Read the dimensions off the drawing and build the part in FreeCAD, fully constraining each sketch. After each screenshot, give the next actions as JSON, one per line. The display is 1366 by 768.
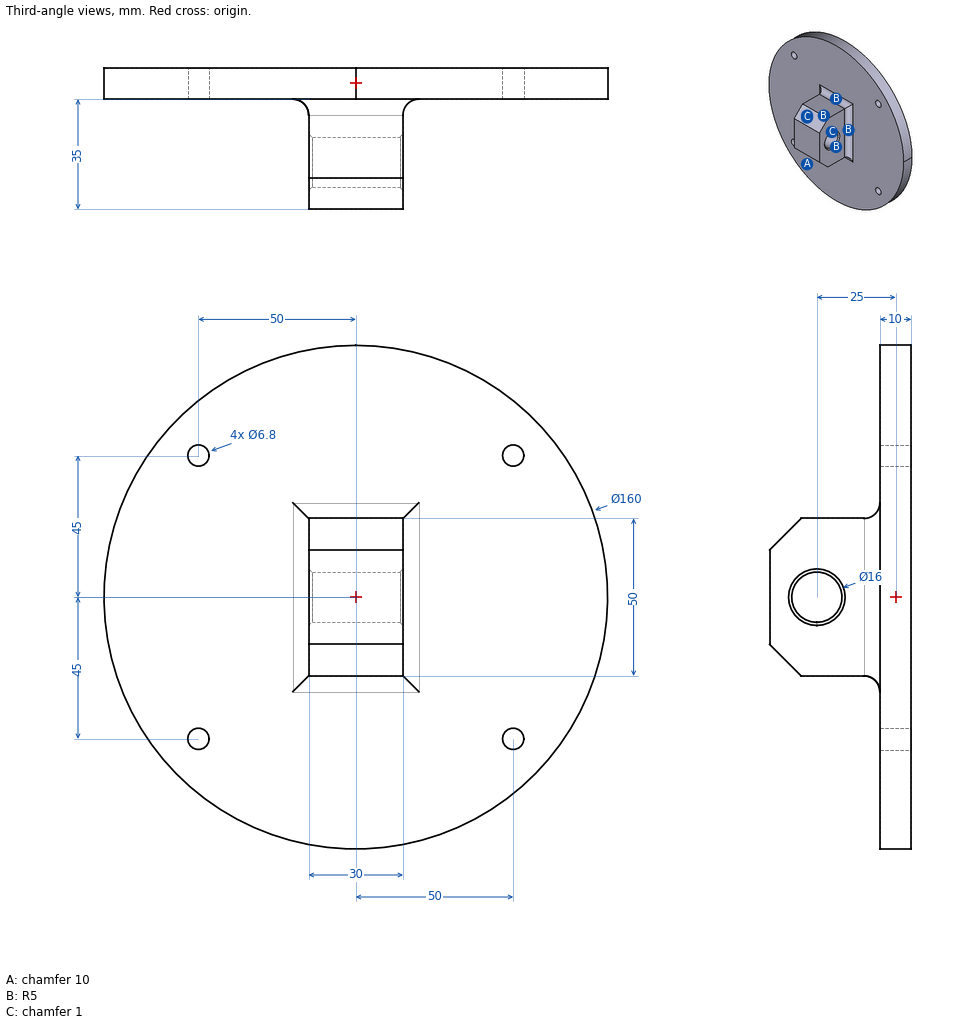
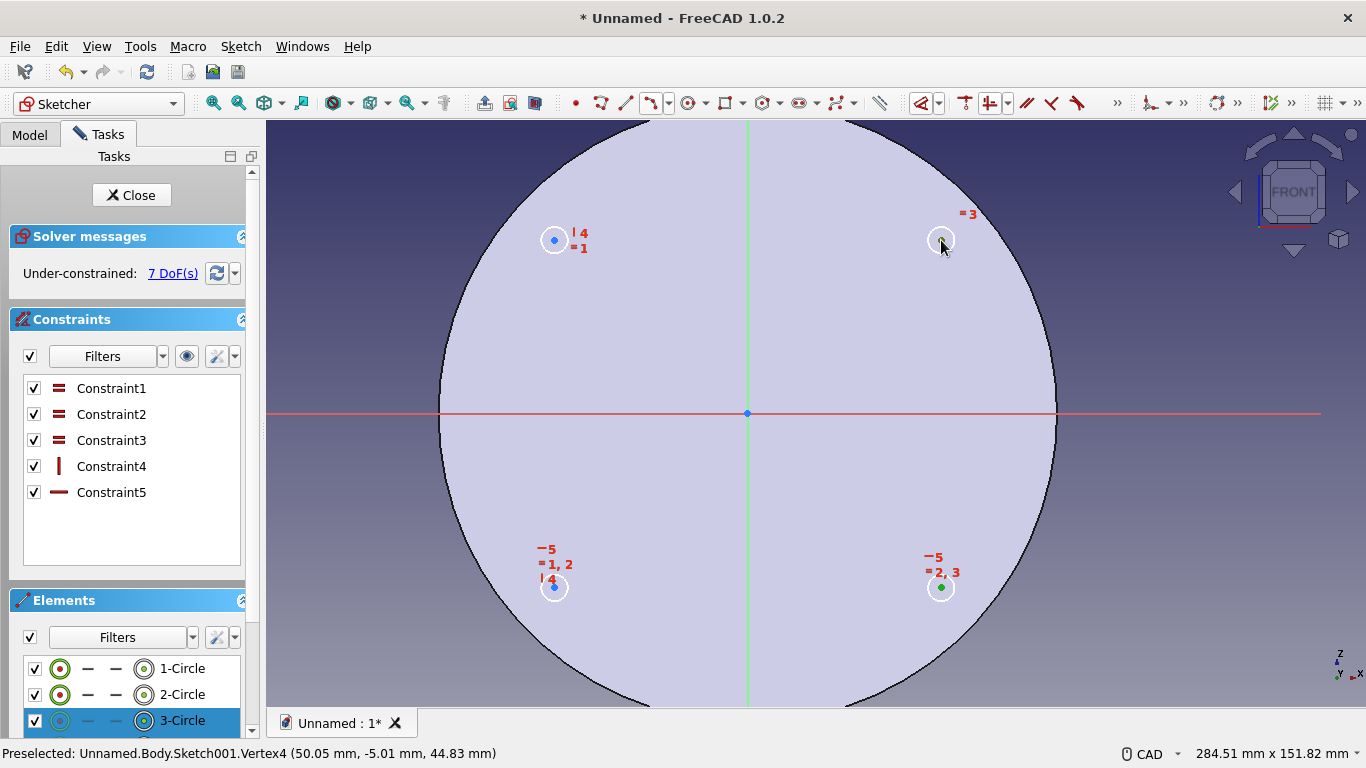
{"action": "left_click", "coordinate": [1008, 104]}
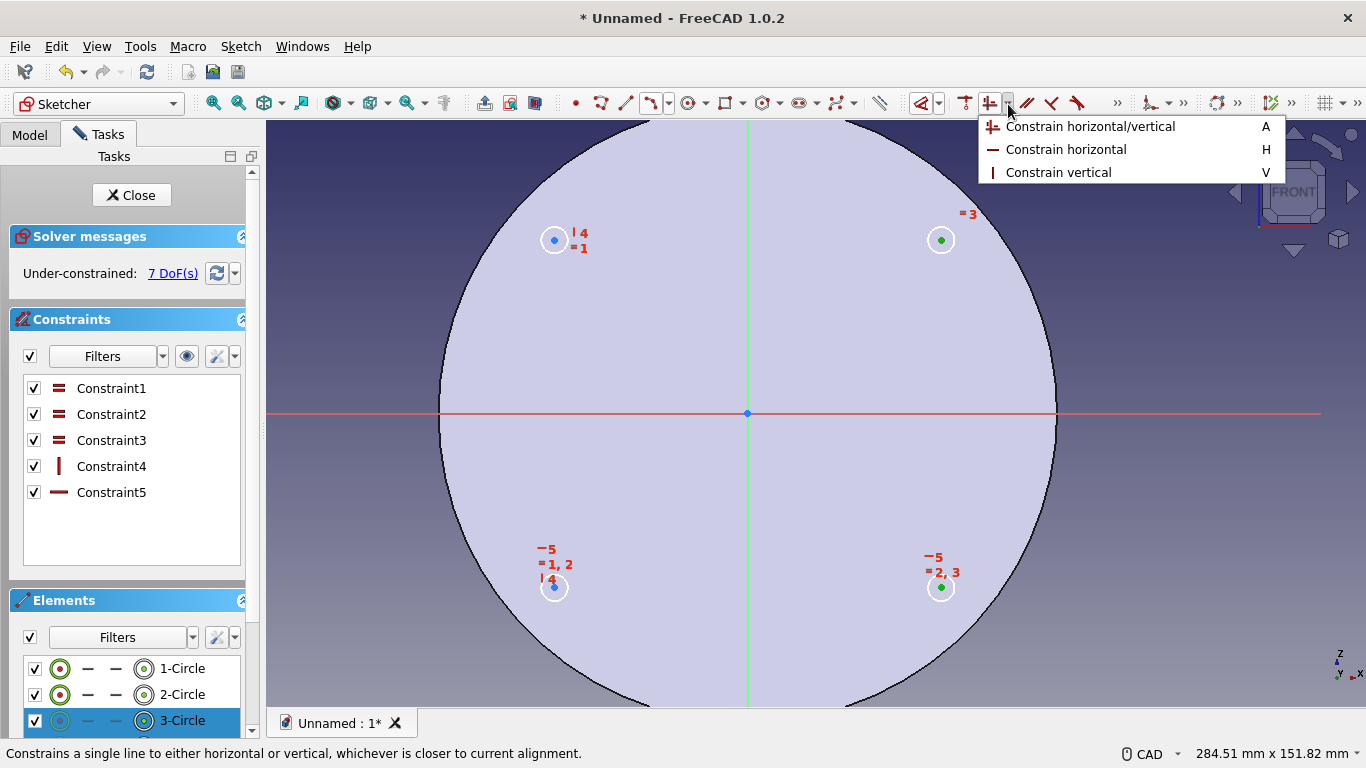
{"action": "left_click", "coordinate": [1132, 172]}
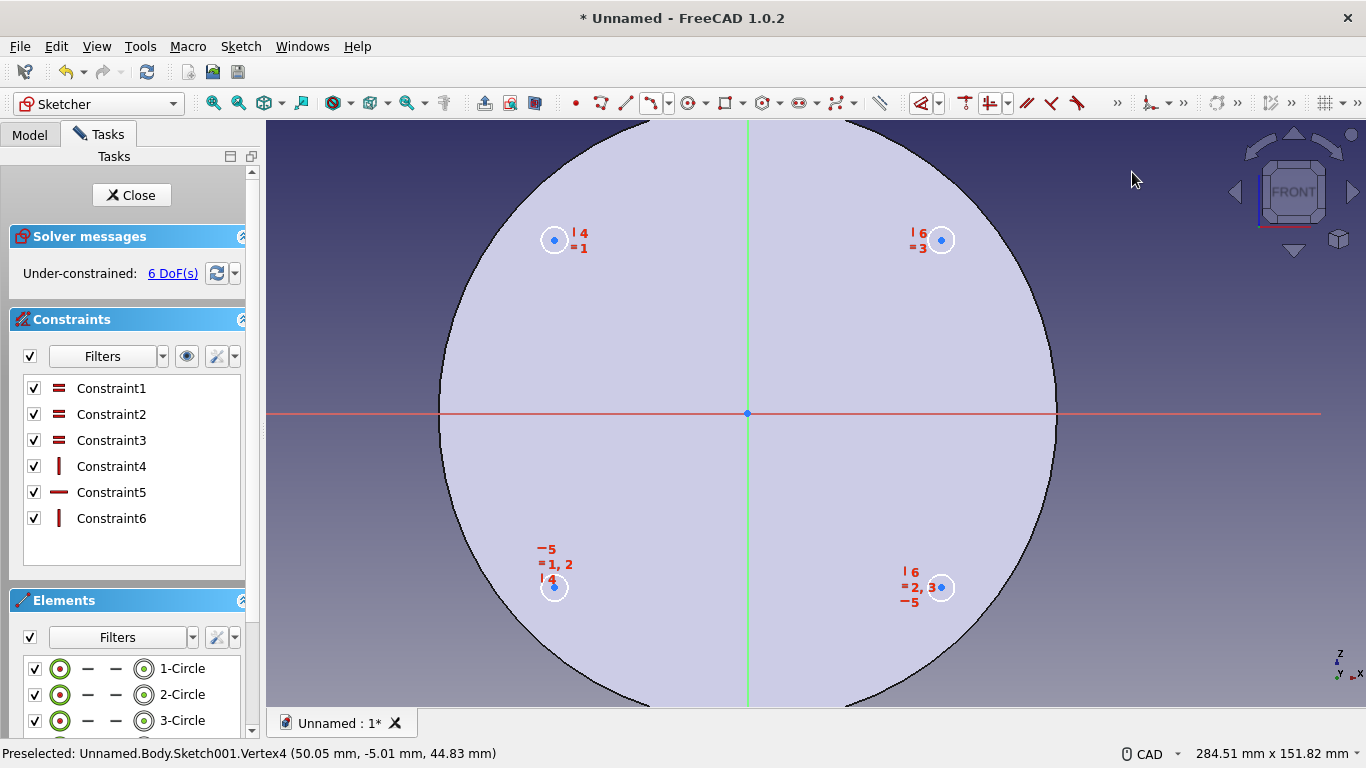
{"action": "left_click", "coordinate": [555, 240]}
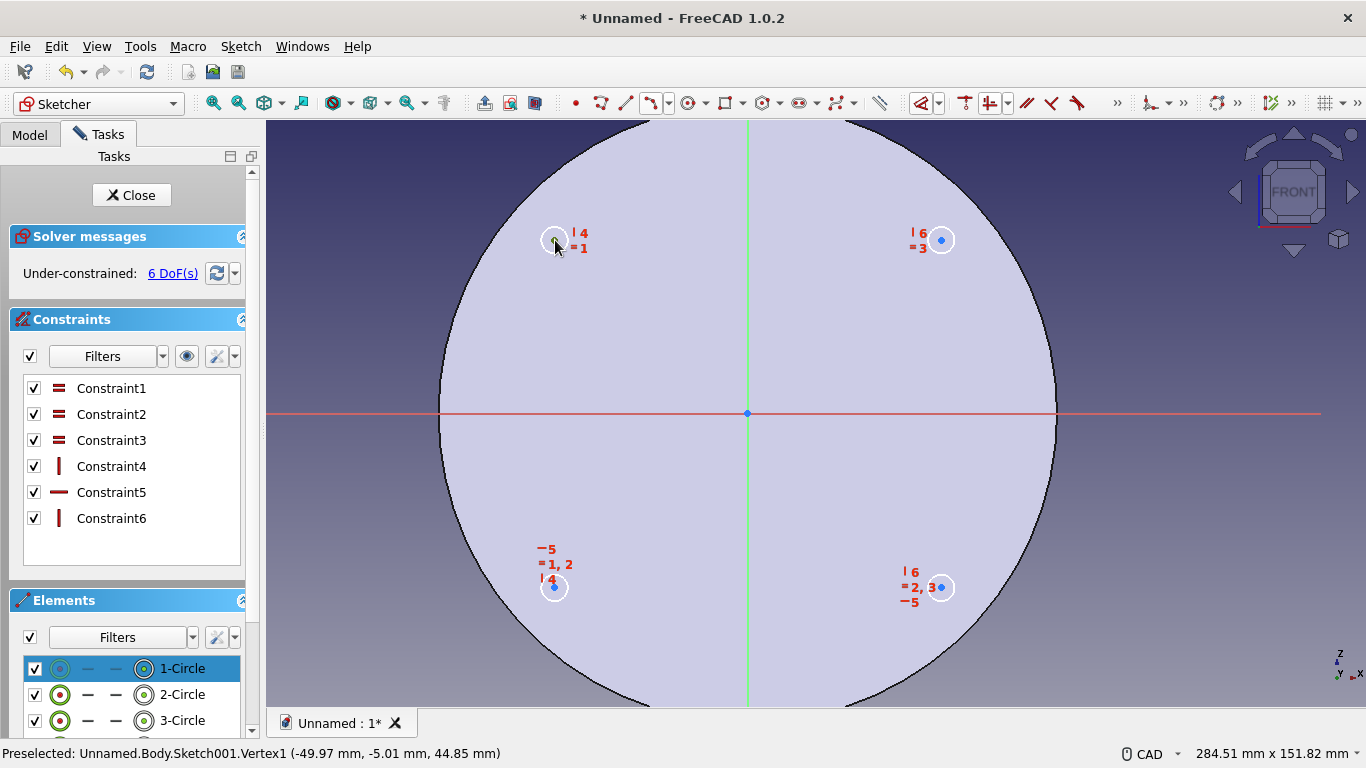
{"action": "left_click", "coordinate": [941, 240]}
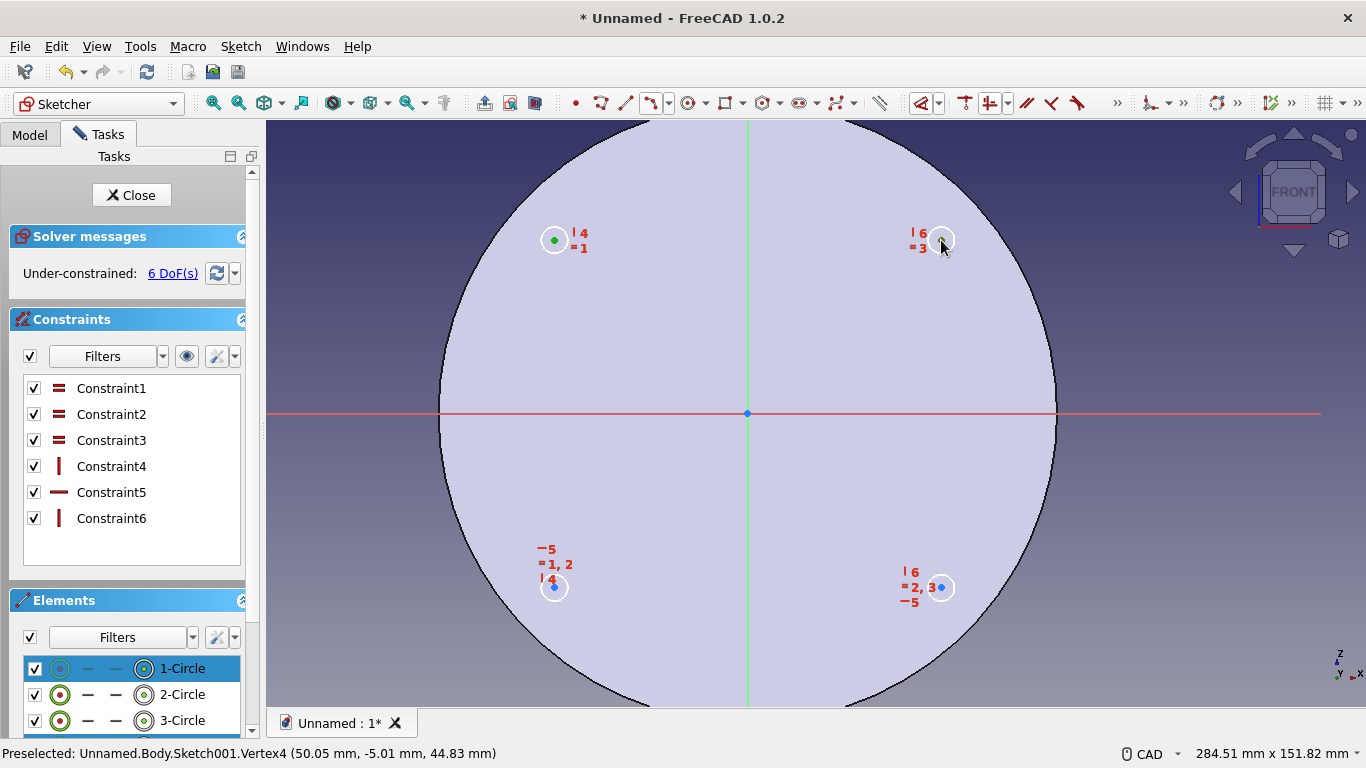
{"action": "key", "text": "h"}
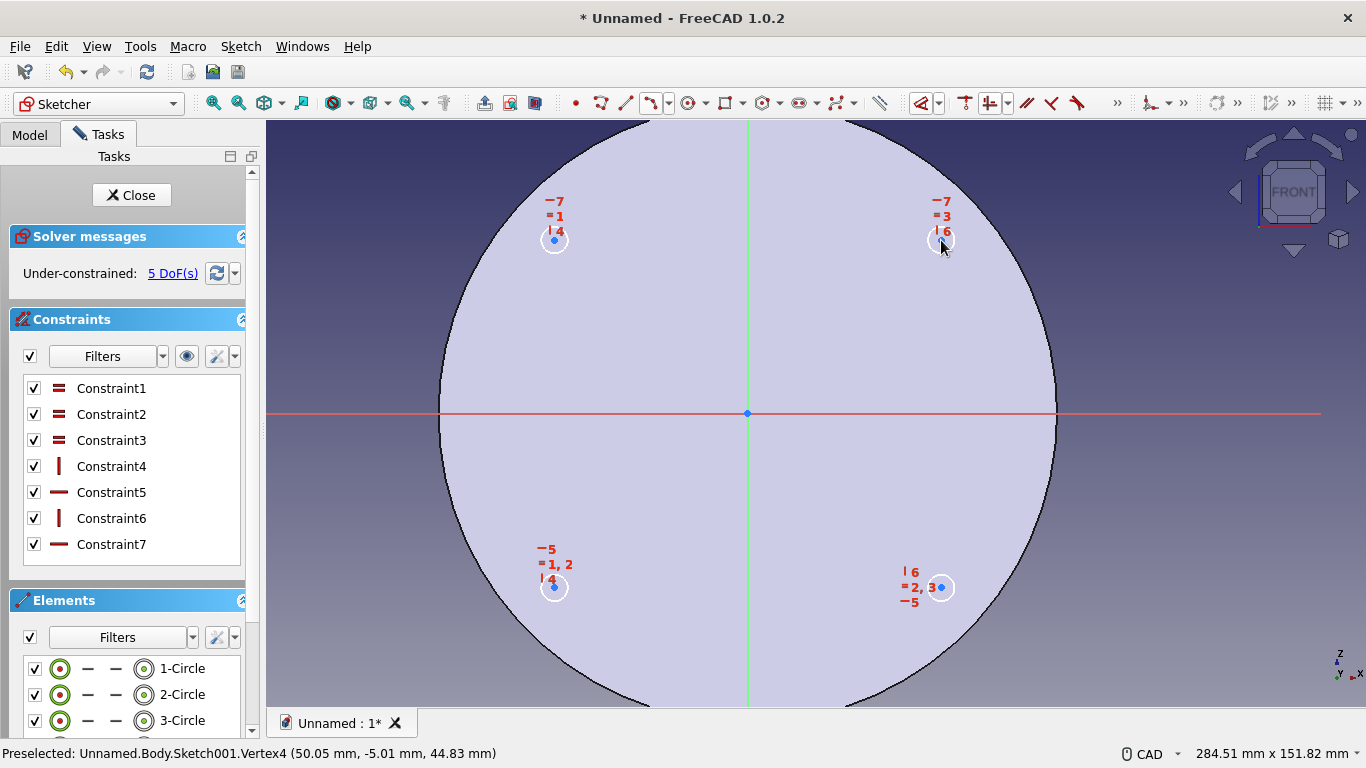
{"action": "left_click", "coordinate": [920, 104]}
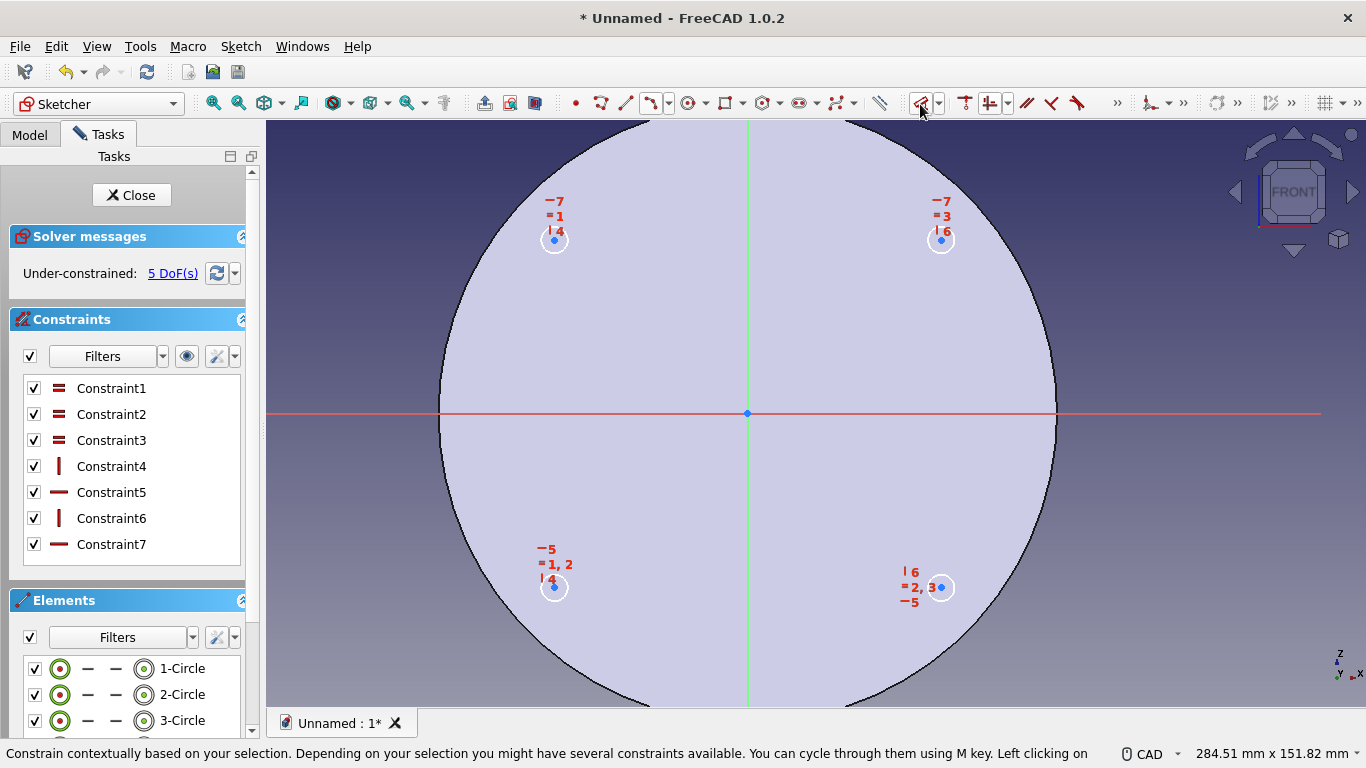
{"action": "scroll", "coordinate": [564, 231], "scroll_direction": "up", "scroll_amount": 3}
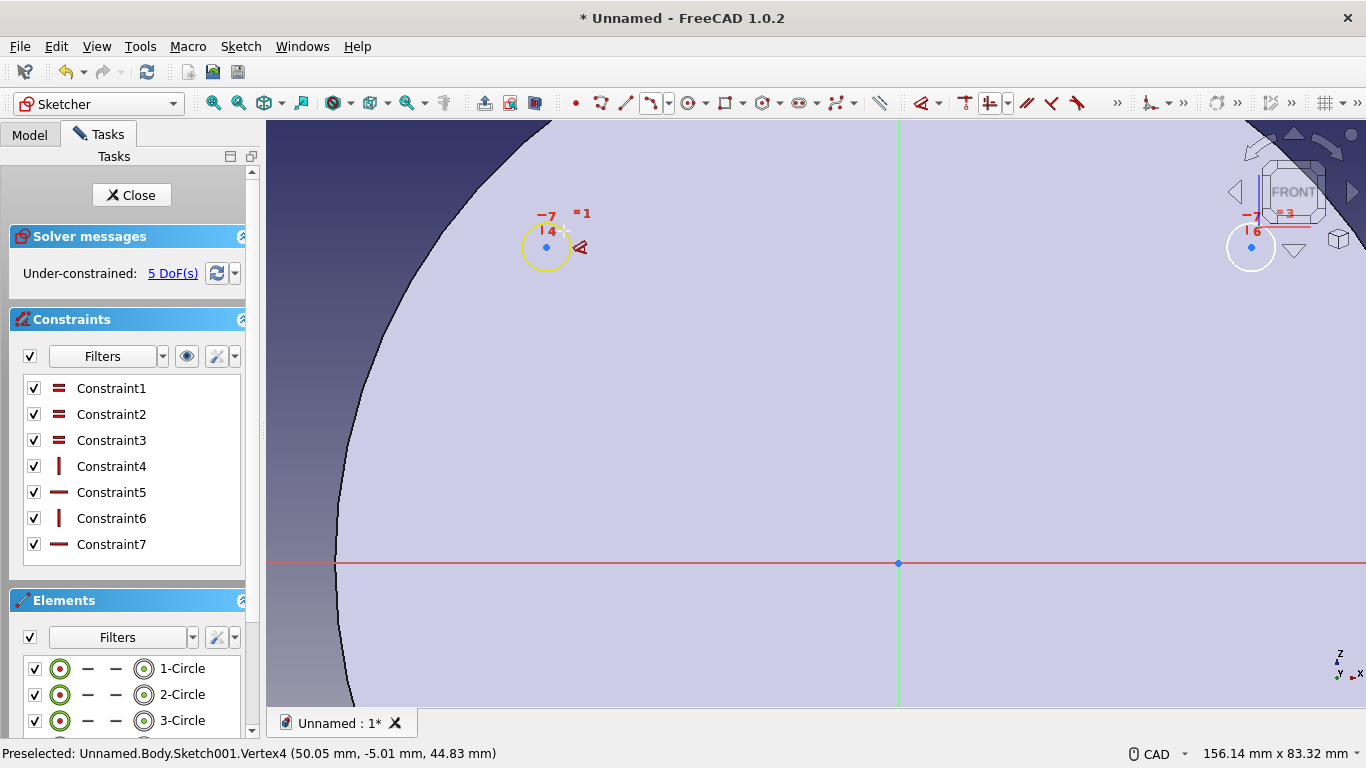
{"action": "left_click", "coordinate": [564, 230]}
{"action": "left_click", "coordinate": [587, 207]}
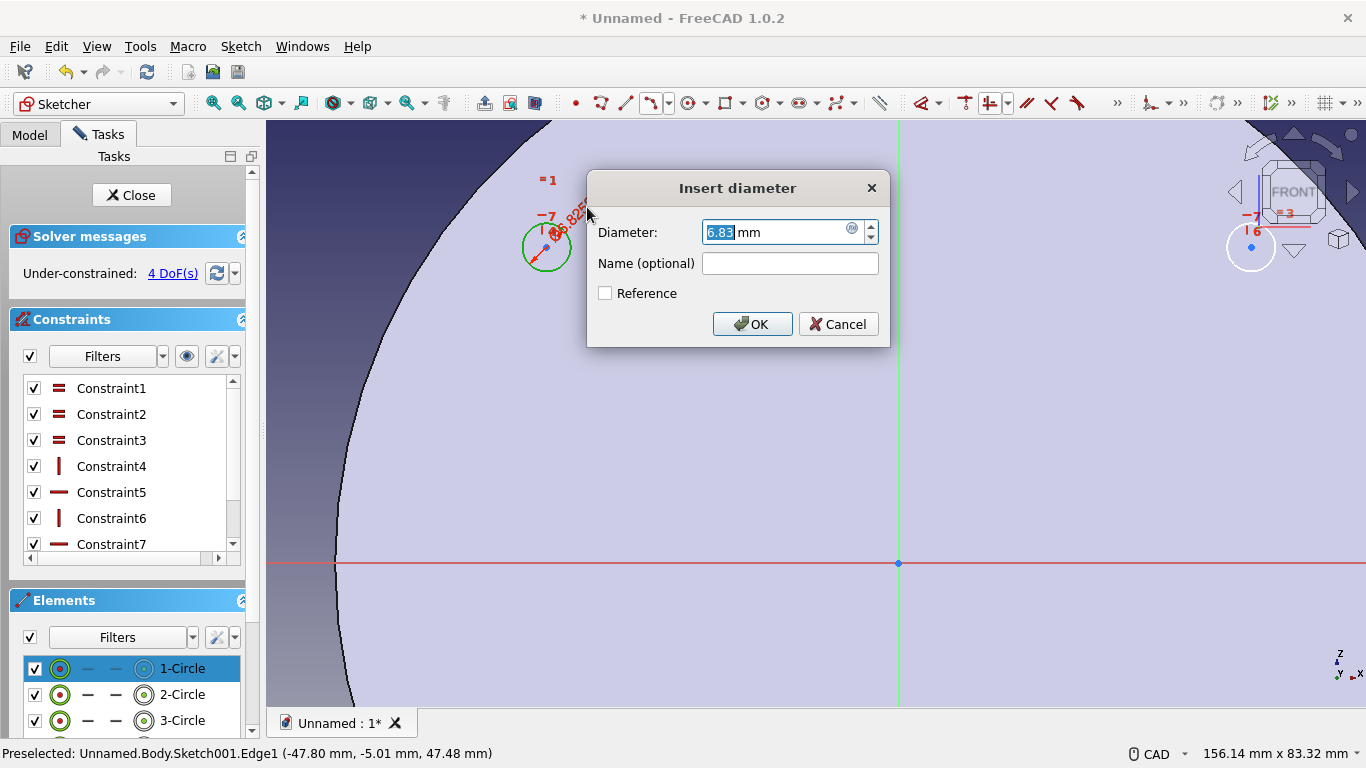
{"action": "type", "text": "6.8"}
{"action": "key", "text": "Return"}